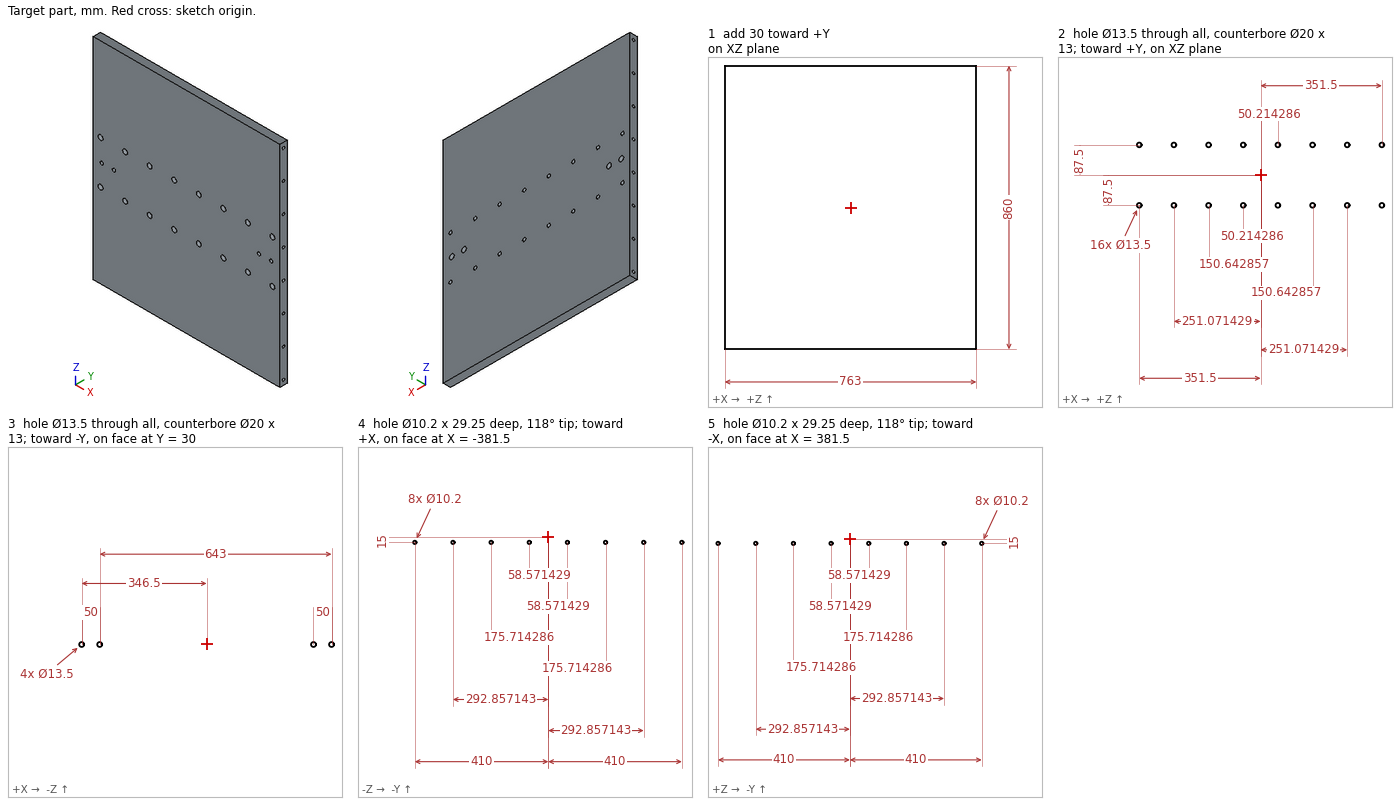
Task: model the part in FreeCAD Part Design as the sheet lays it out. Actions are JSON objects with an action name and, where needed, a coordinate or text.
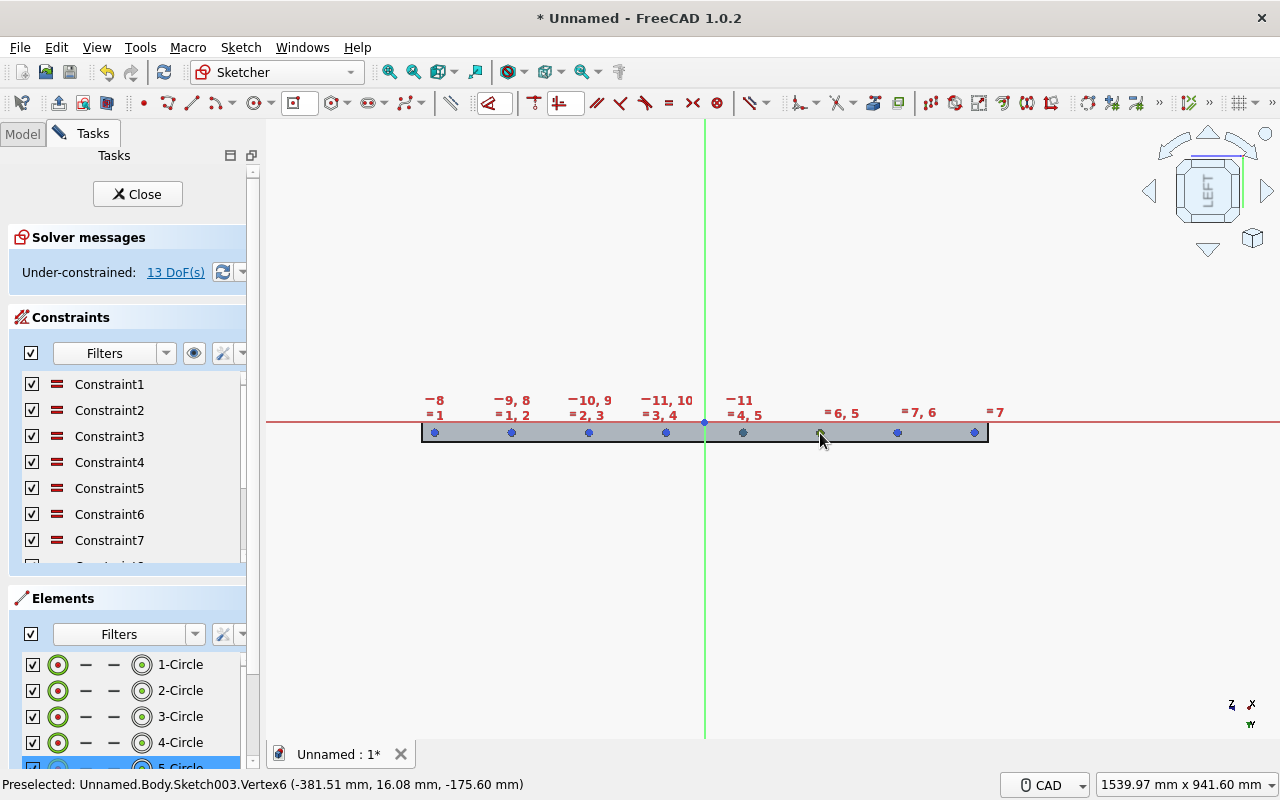
{"action": "left_click", "coordinate": [578, 104]}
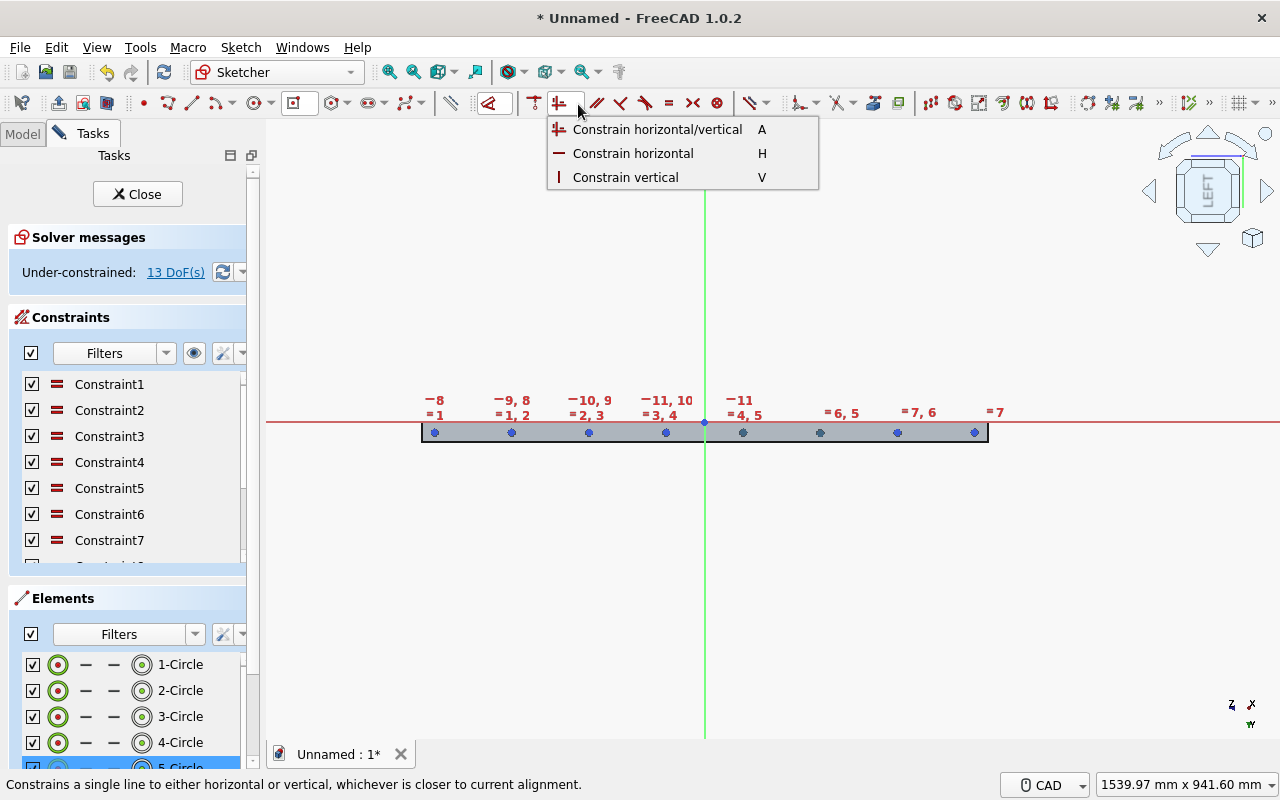
{"action": "left_click", "coordinate": [683, 153]}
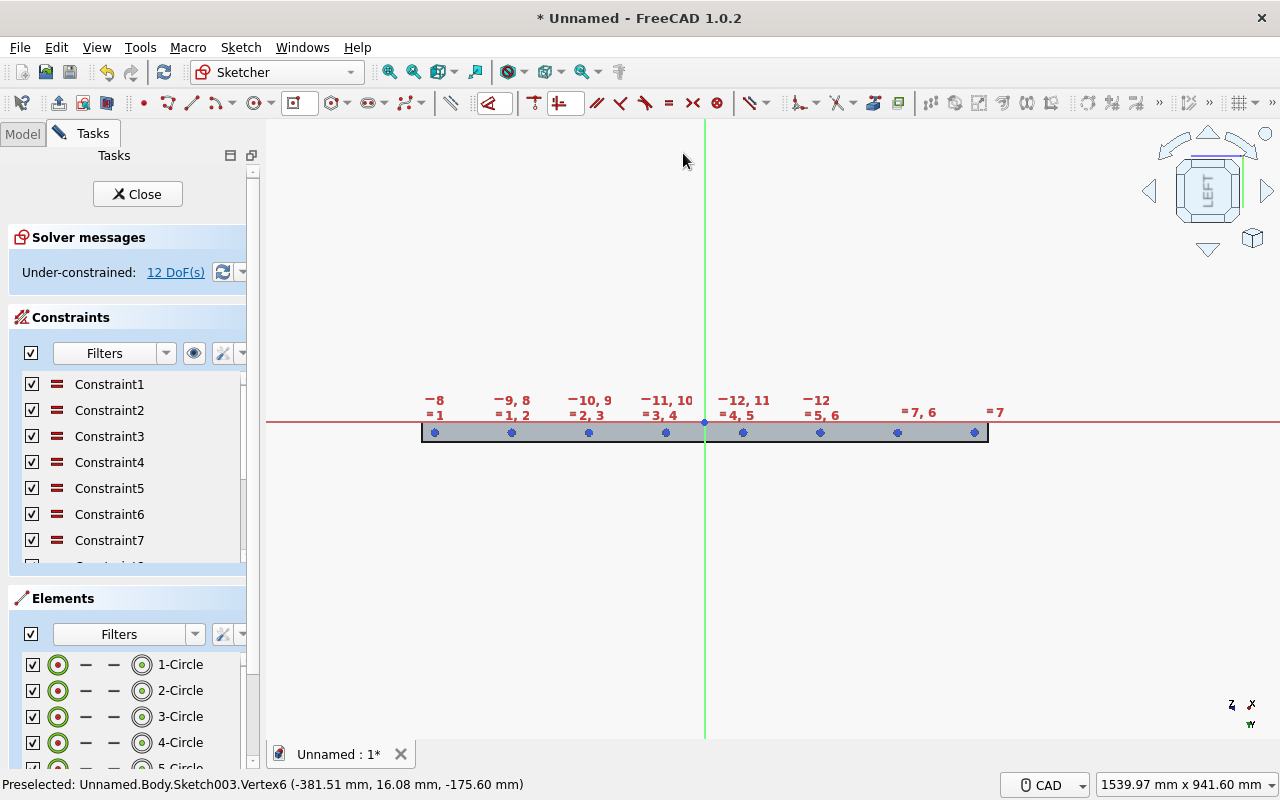
{"action": "left_click", "coordinate": [820, 433]}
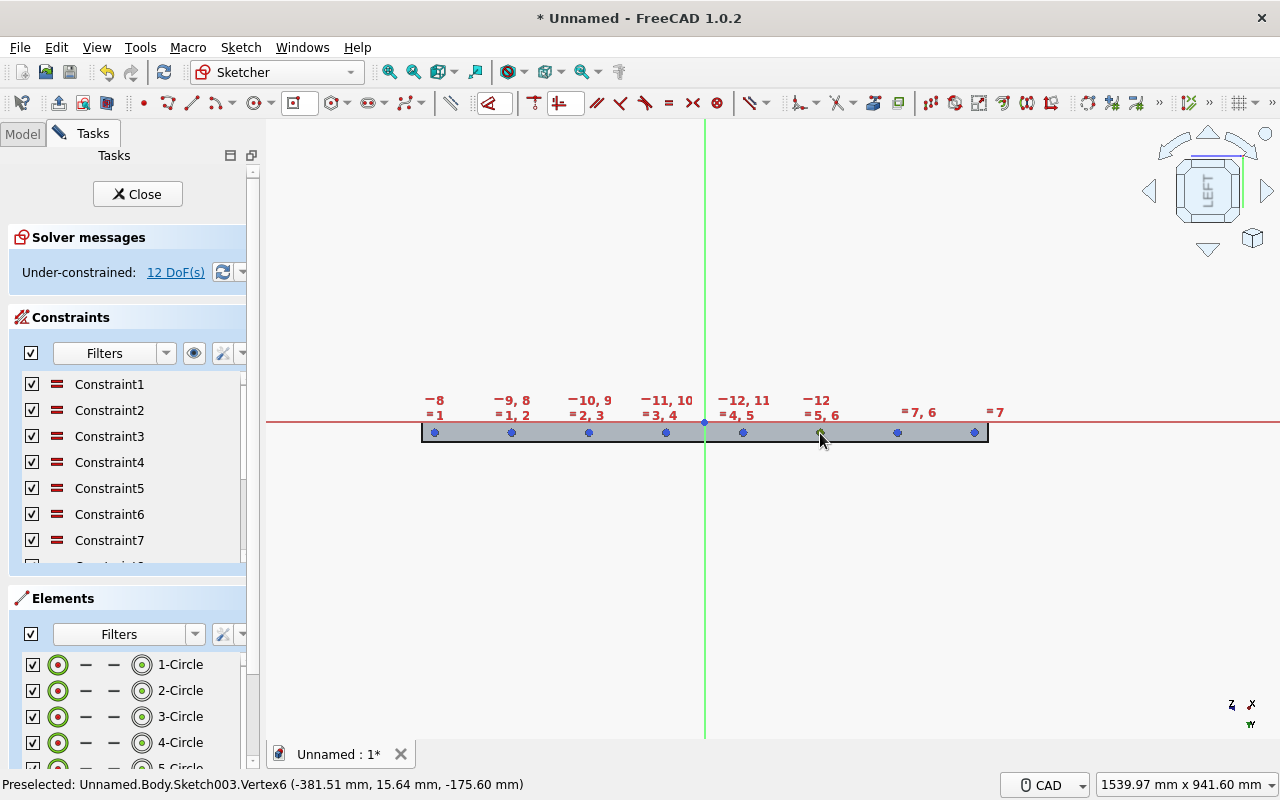
{"action": "left_click", "coordinate": [898, 433]}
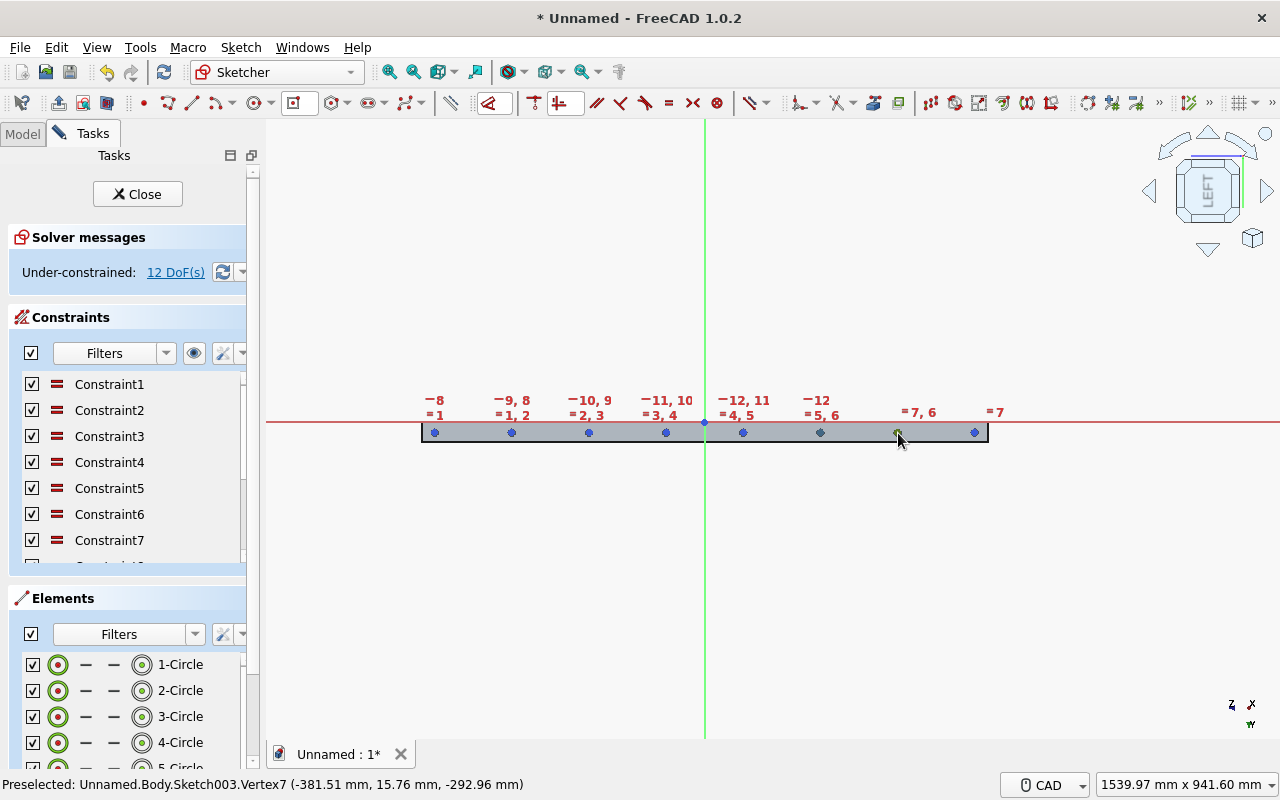
{"action": "left_click", "coordinate": [578, 104]}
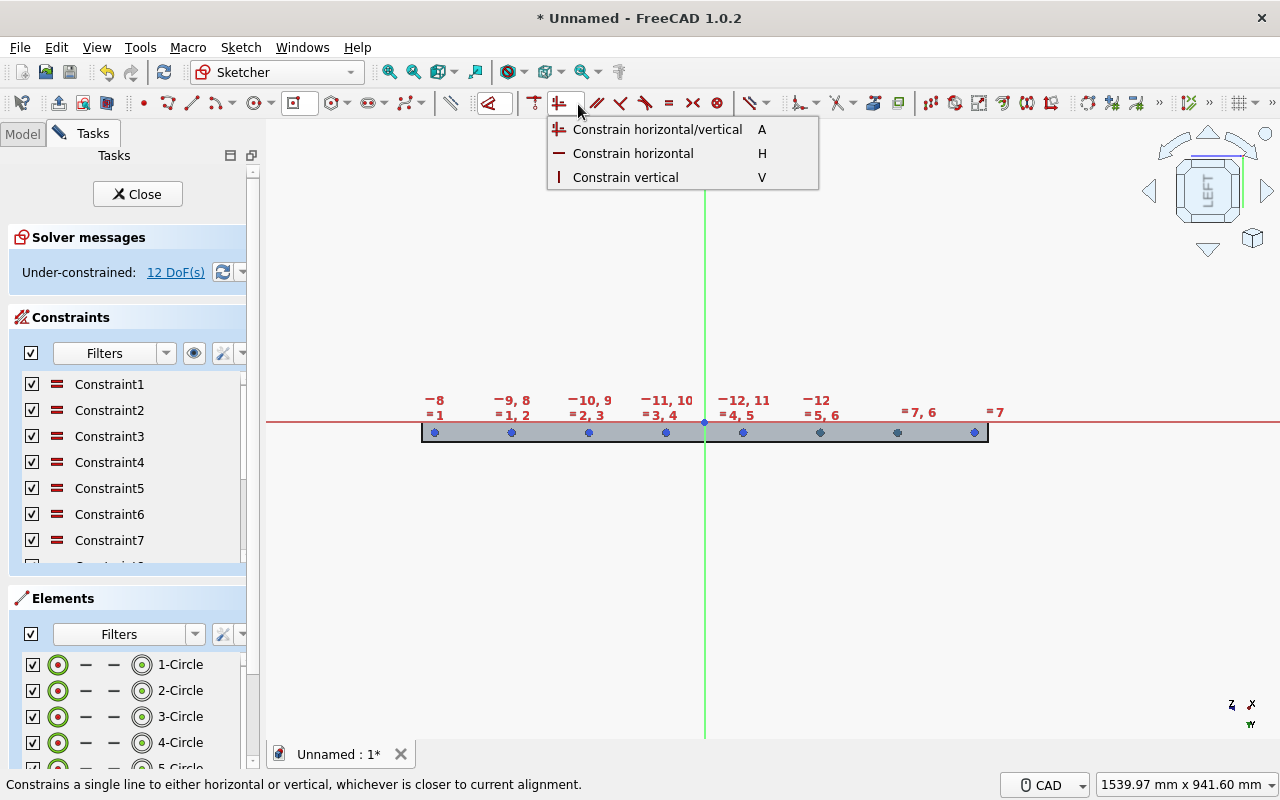
{"action": "left_click", "coordinate": [683, 153]}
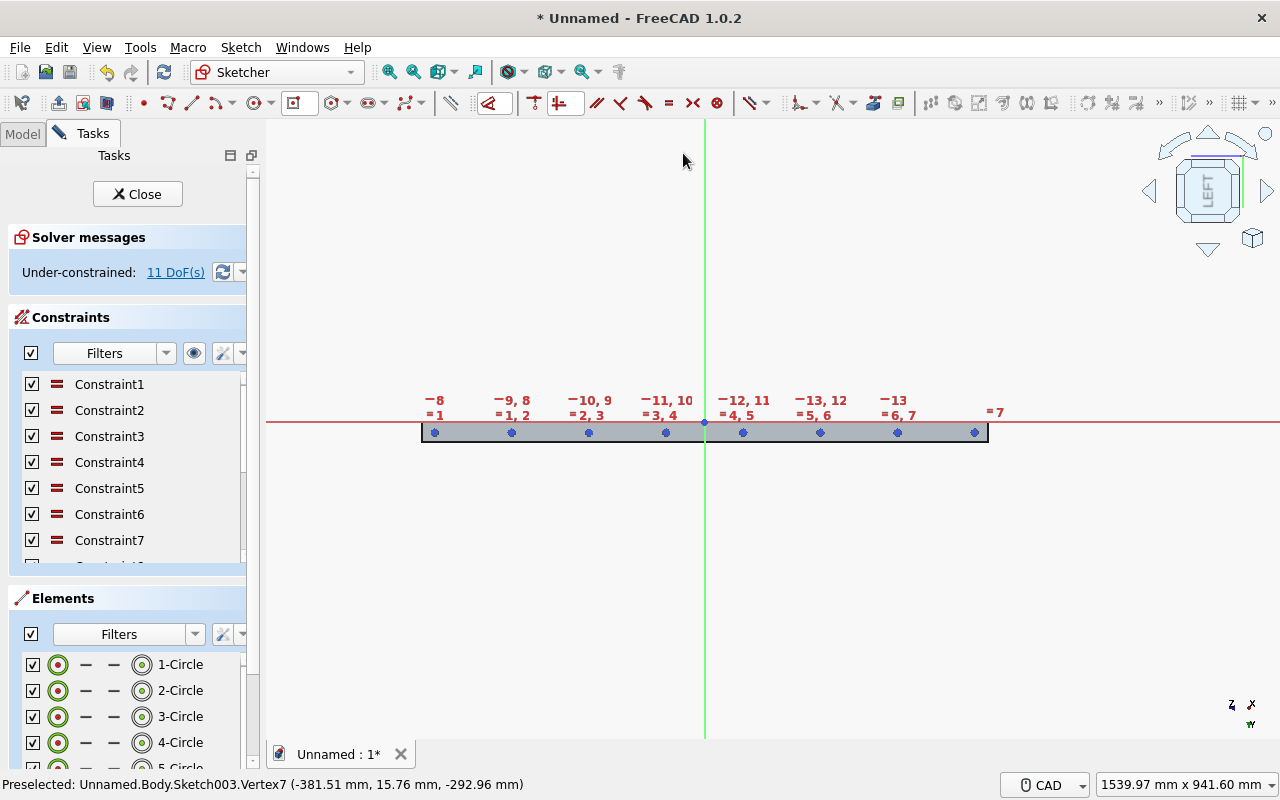
{"action": "left_click", "coordinate": [898, 433]}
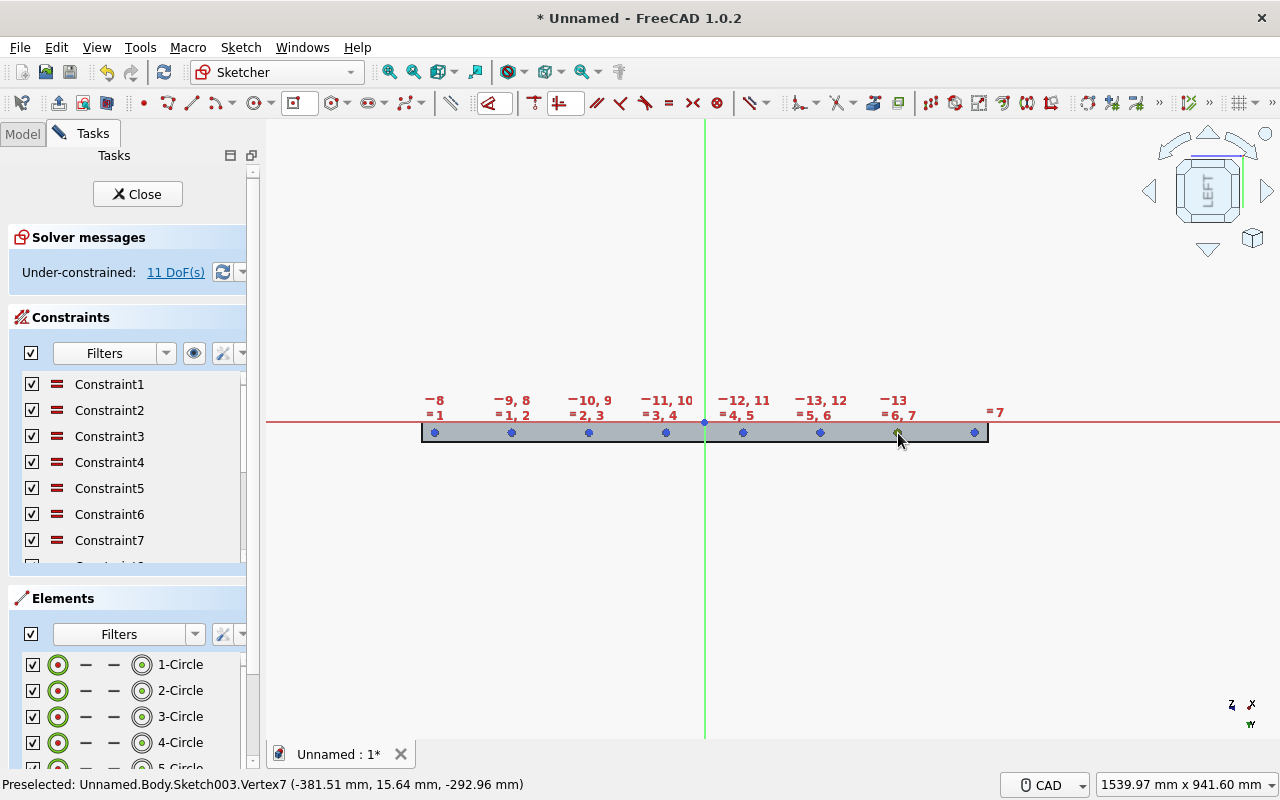
{"action": "left_click", "coordinate": [975, 433]}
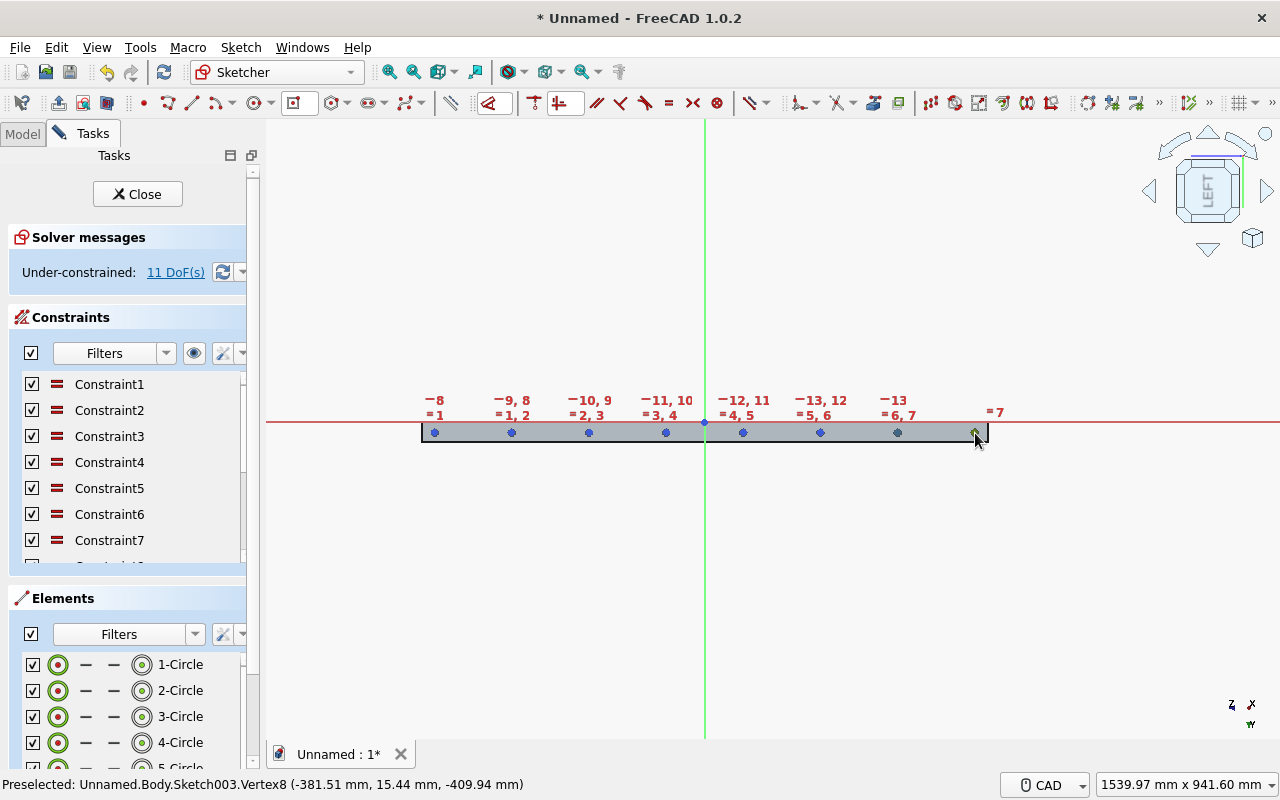
{"action": "key", "text": "h"}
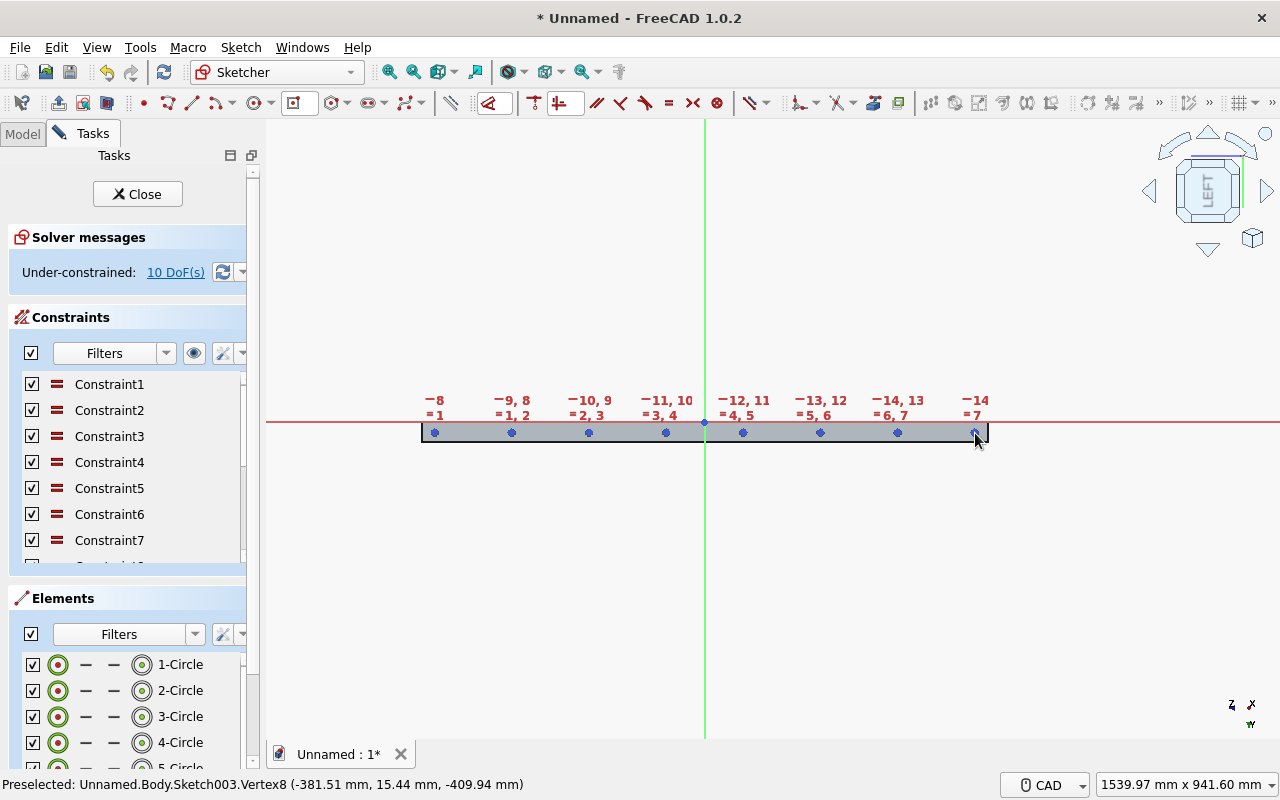
{"action": "scroll", "coordinate": [435, 429], "scroll_direction": "up", "scroll_amount": 9}